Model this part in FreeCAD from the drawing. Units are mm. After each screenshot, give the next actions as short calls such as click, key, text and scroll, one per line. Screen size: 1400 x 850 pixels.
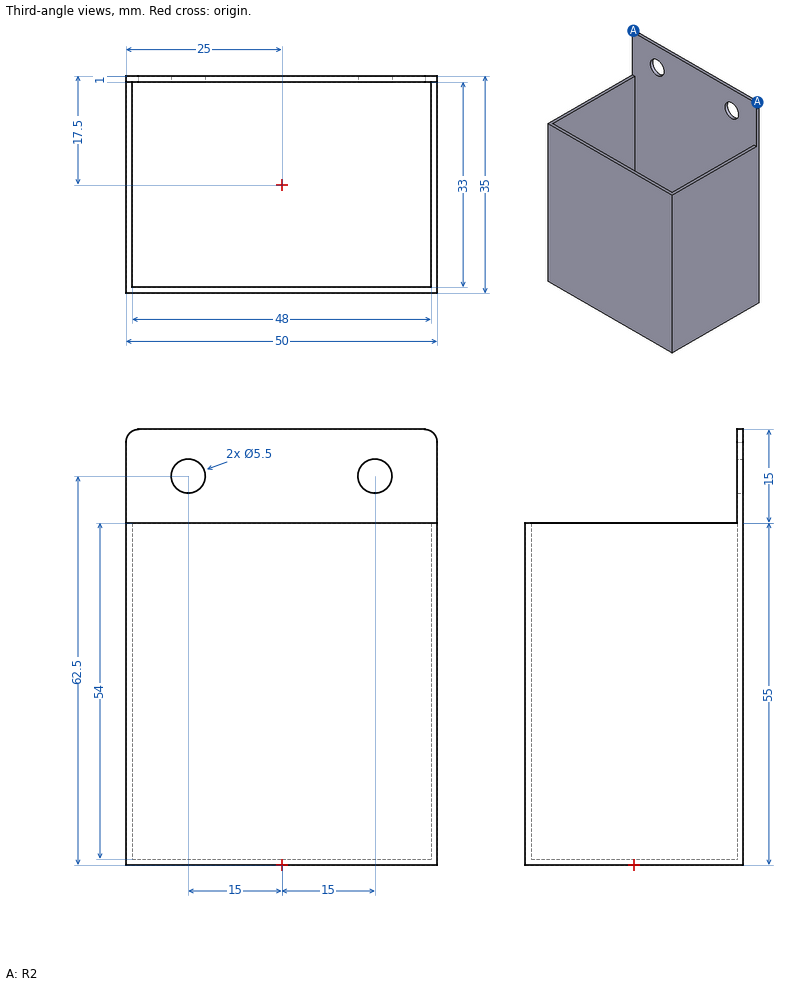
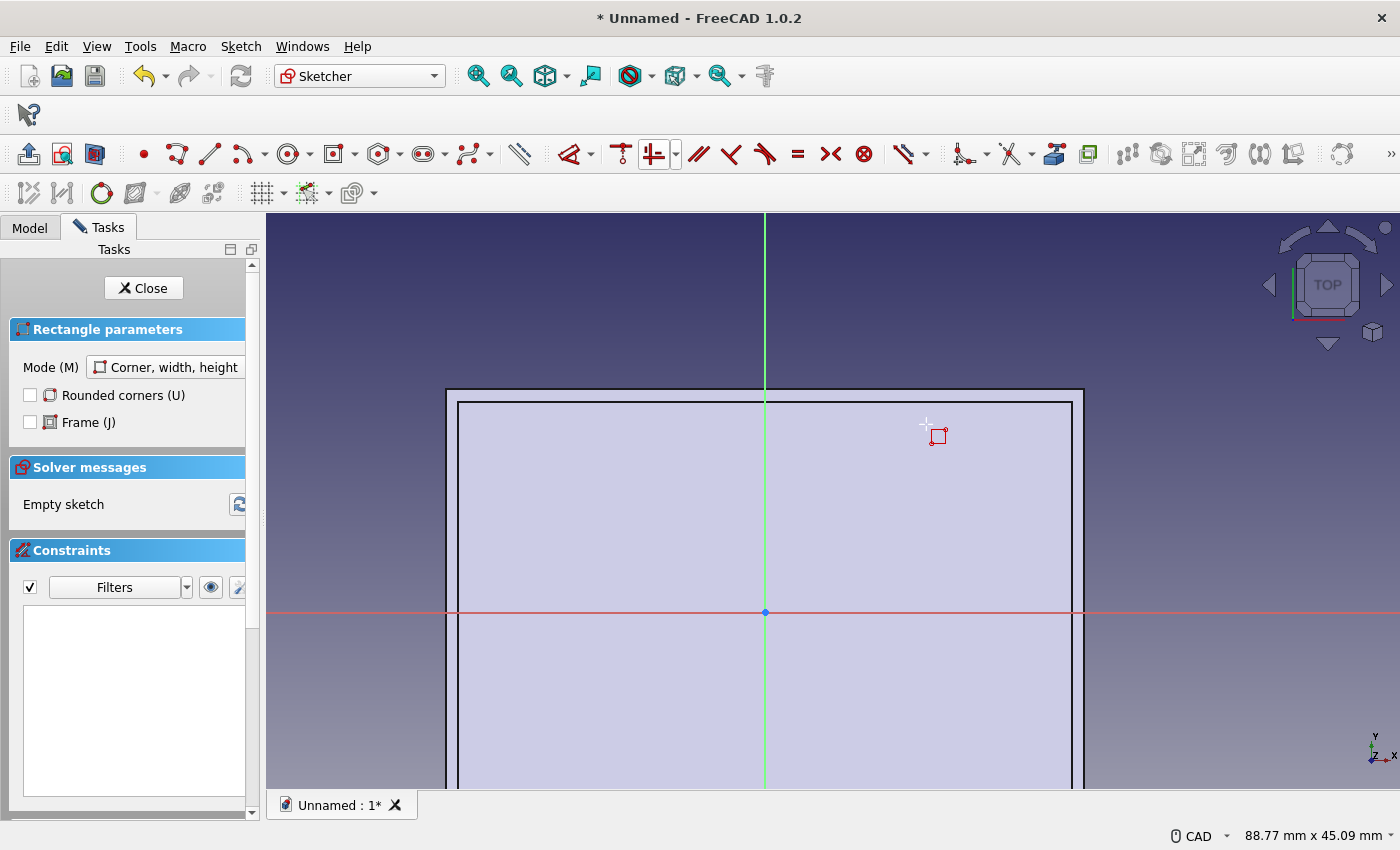
scroll(446, 389, up, 2)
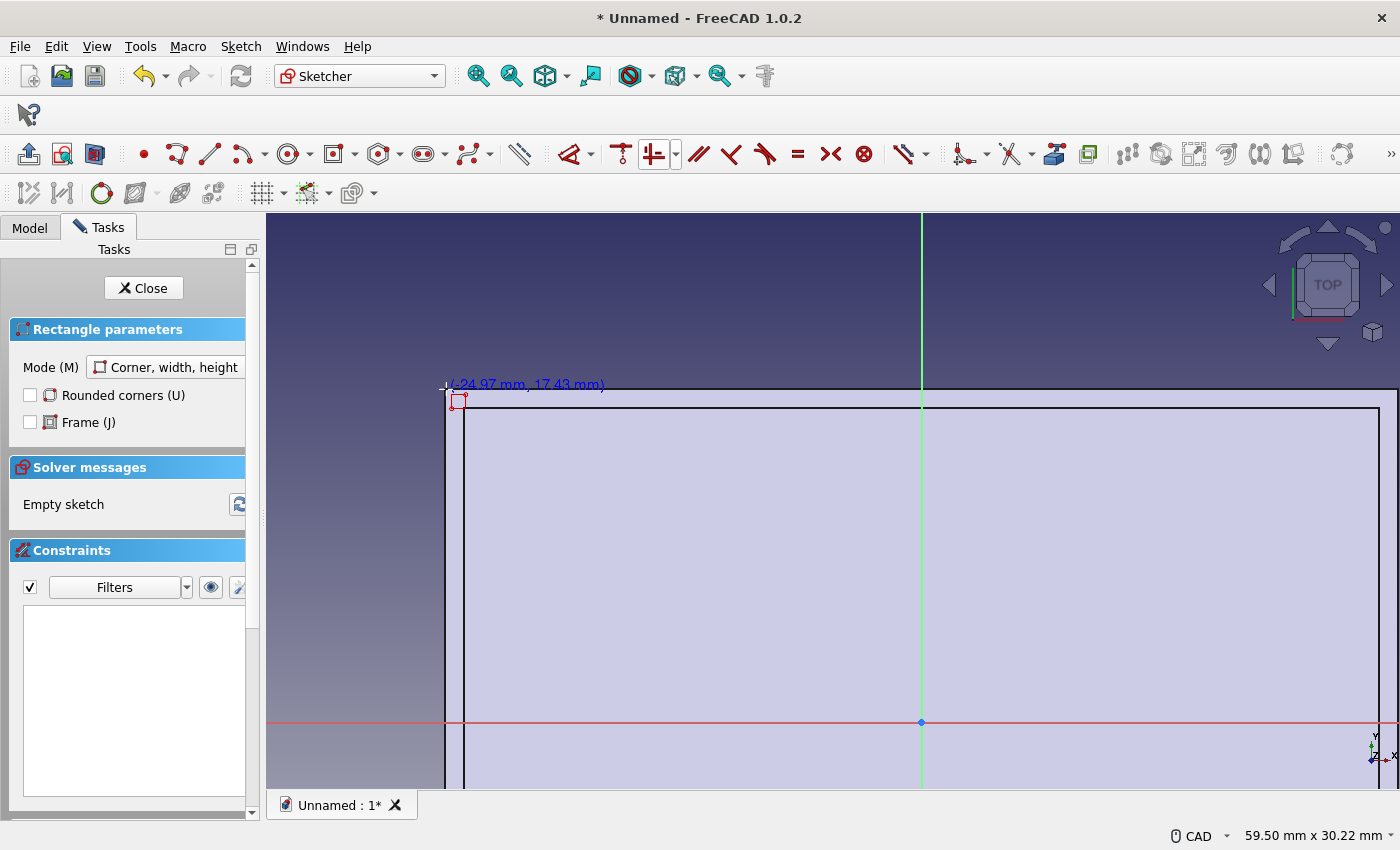
click(445, 389)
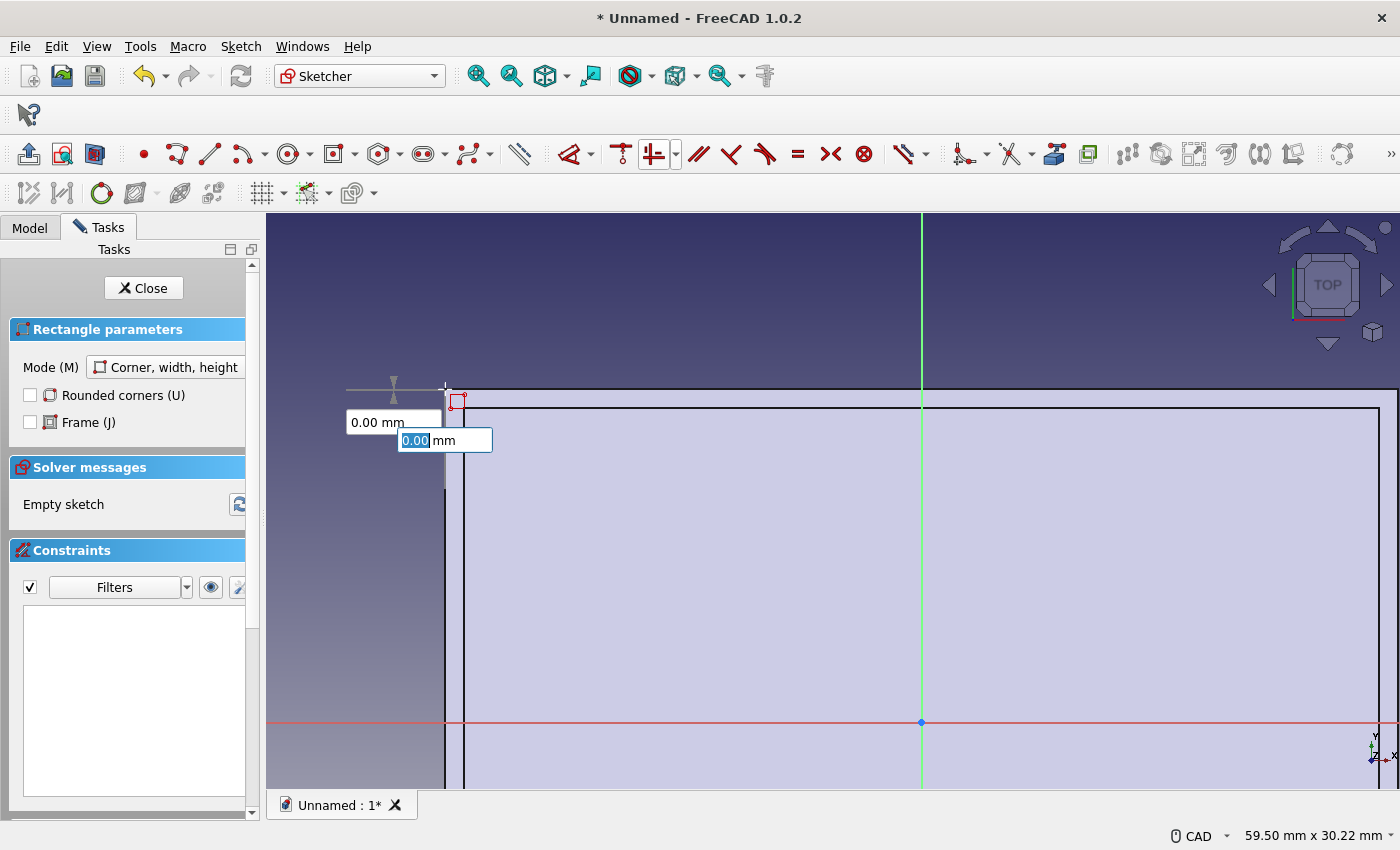
scroll(445, 390, down, 2)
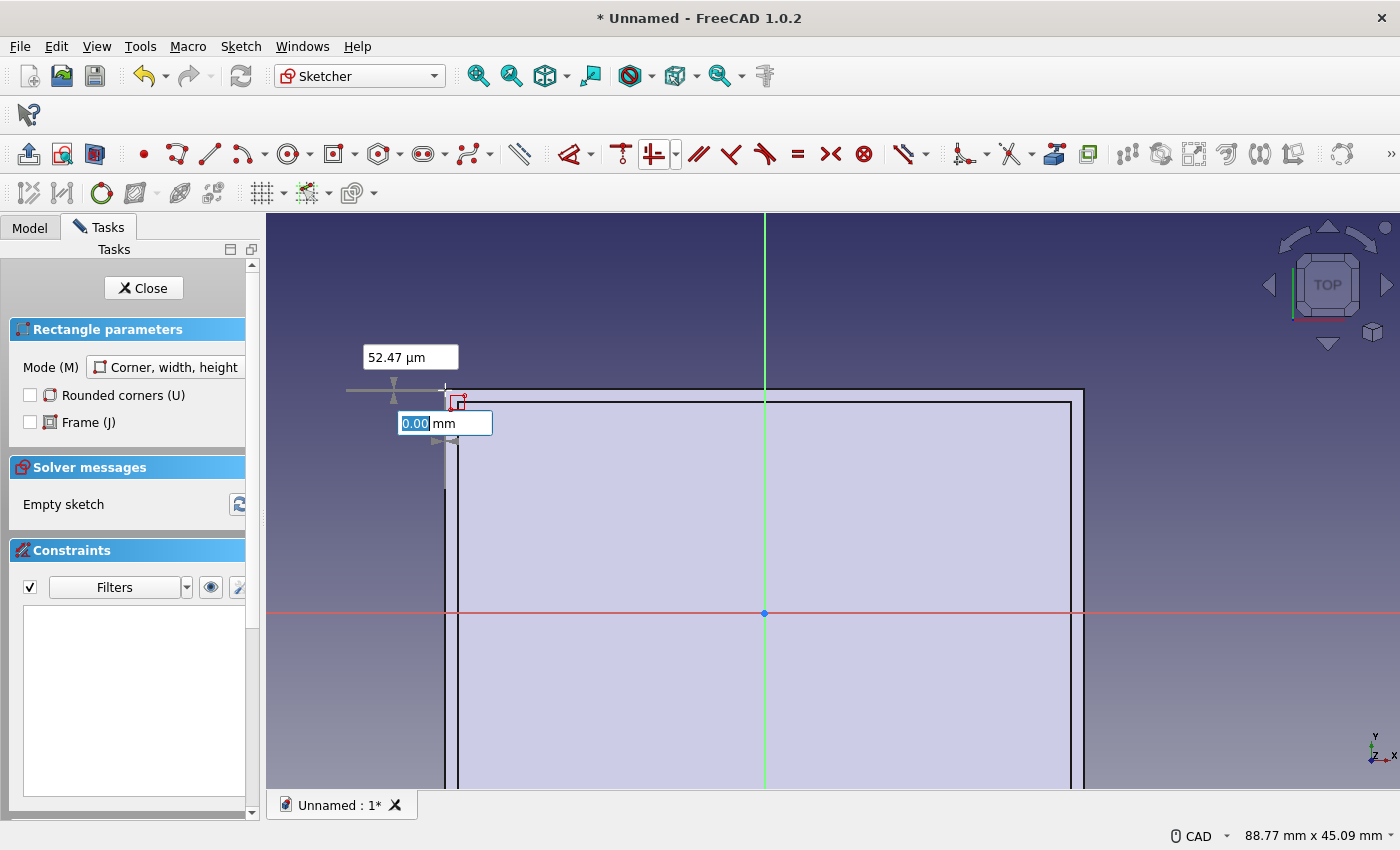
click(1084, 402)
key(Escape)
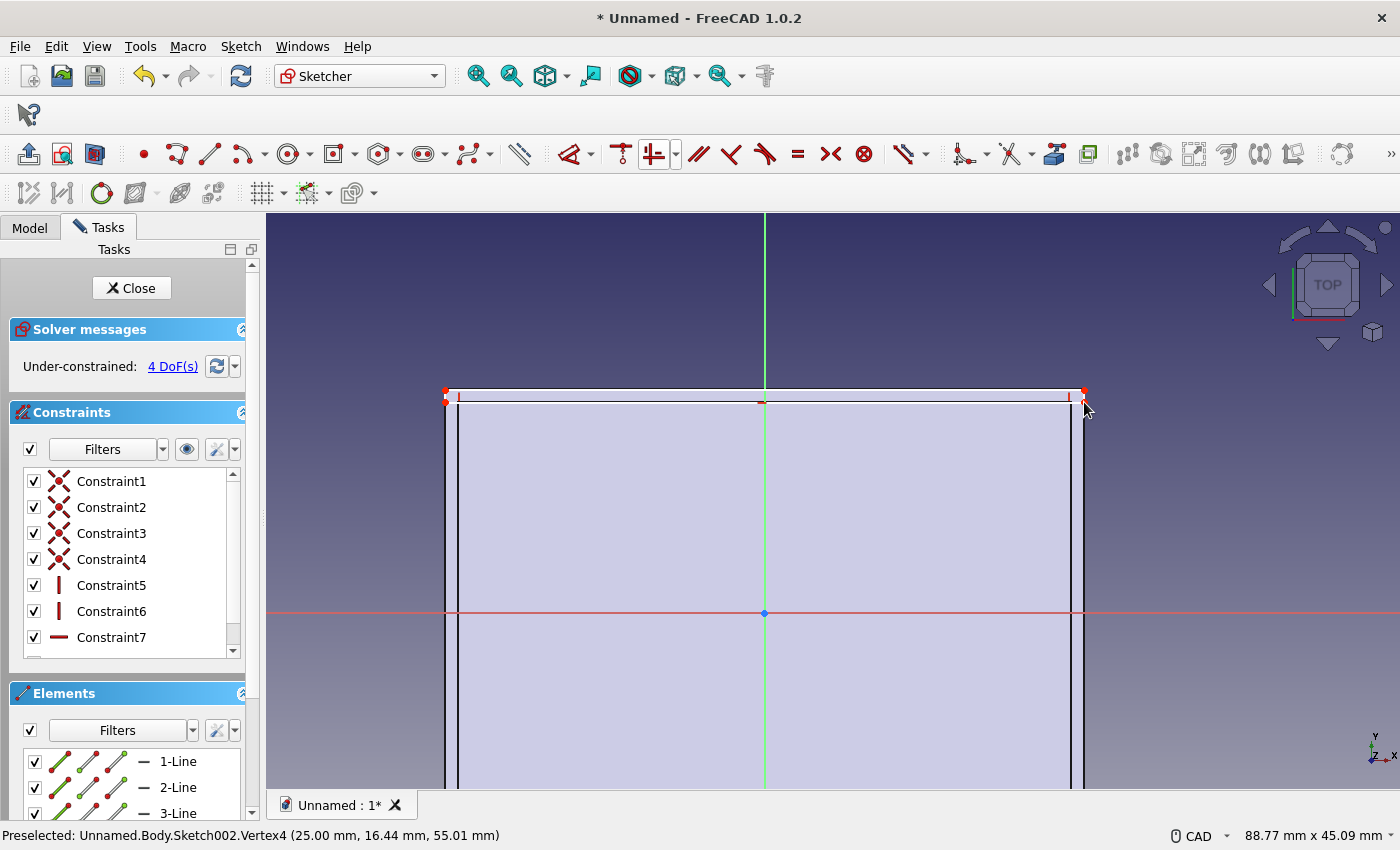
key(d)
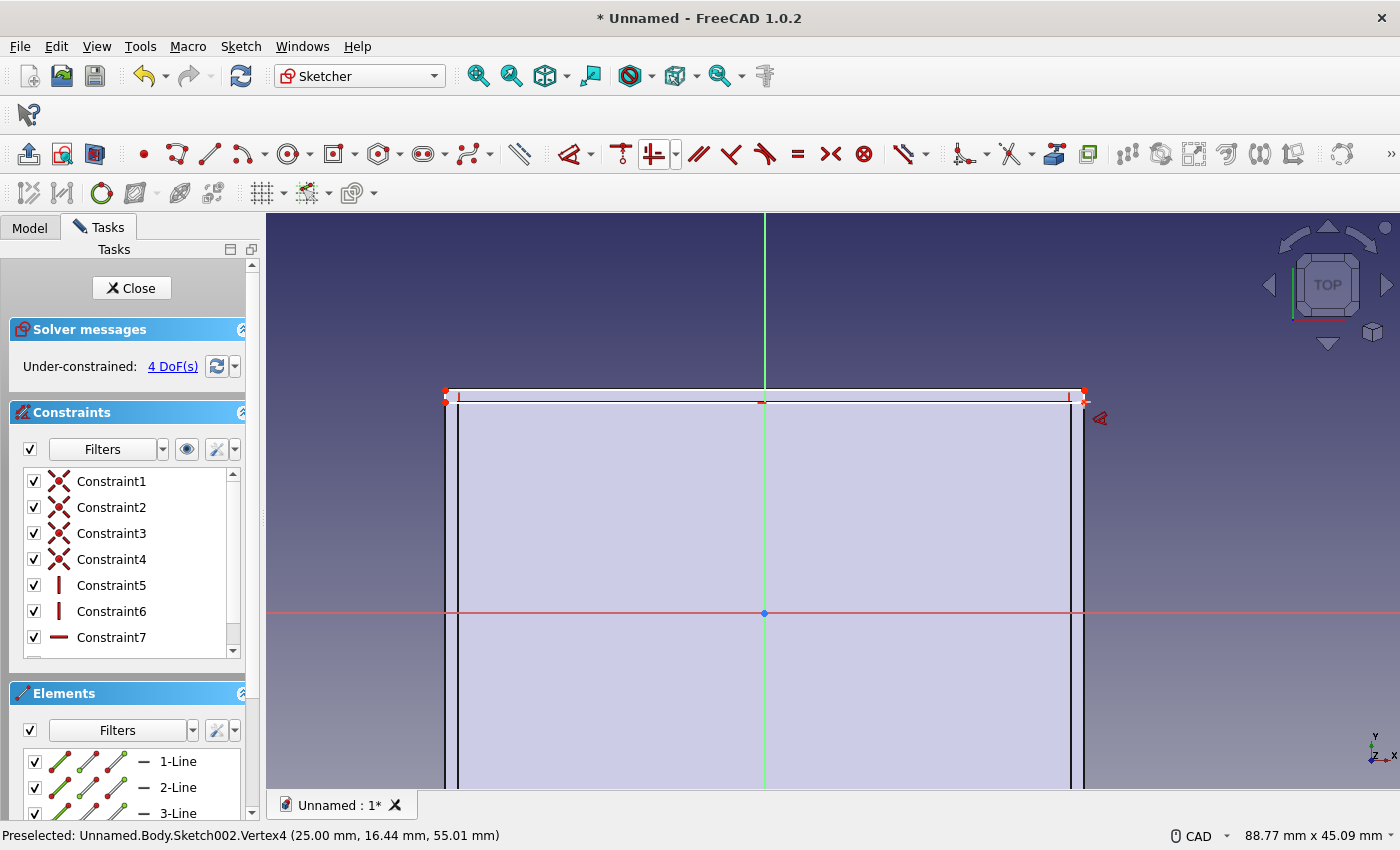
scroll(445, 397, up, 6)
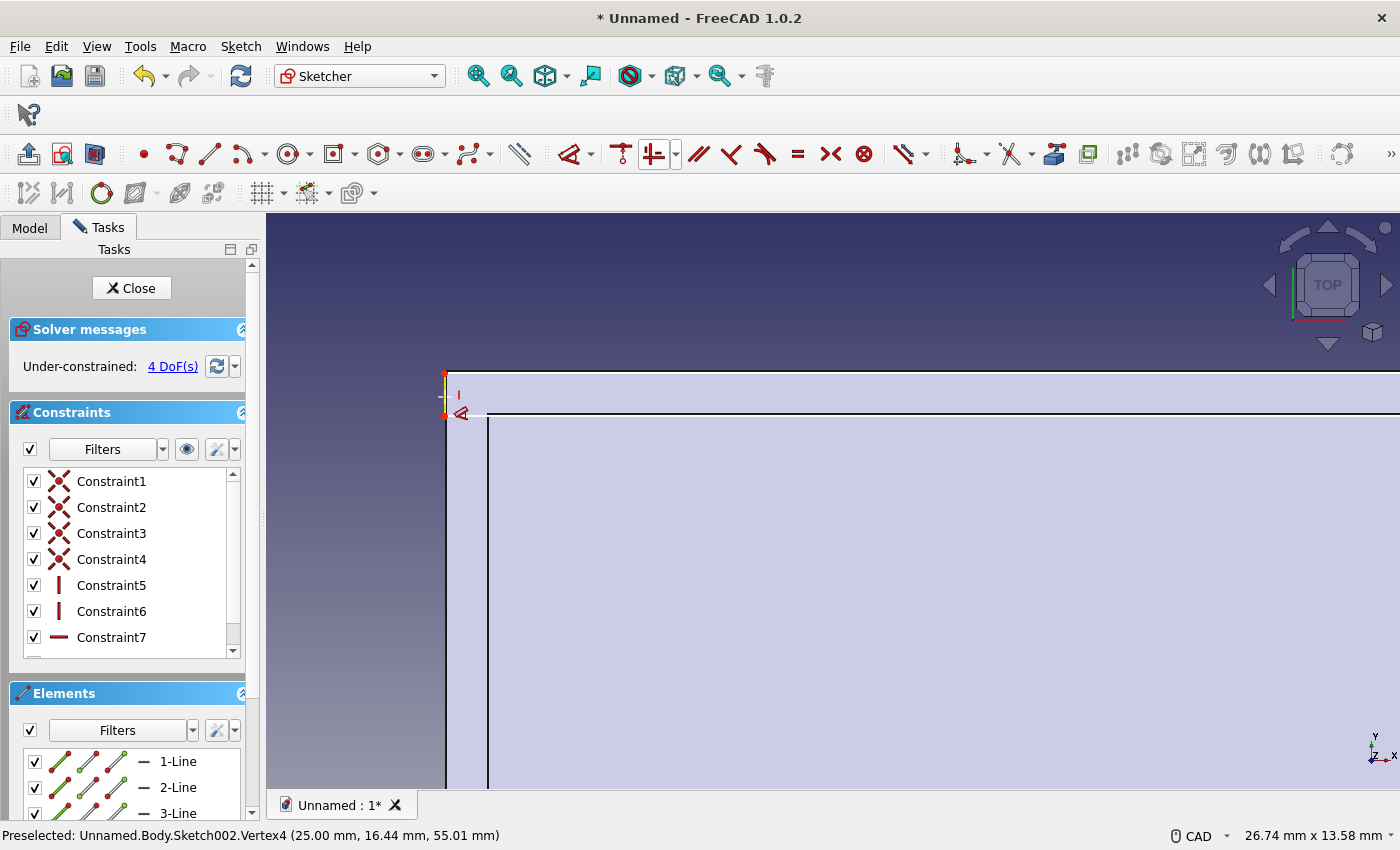
click(445, 395)
click(411, 395)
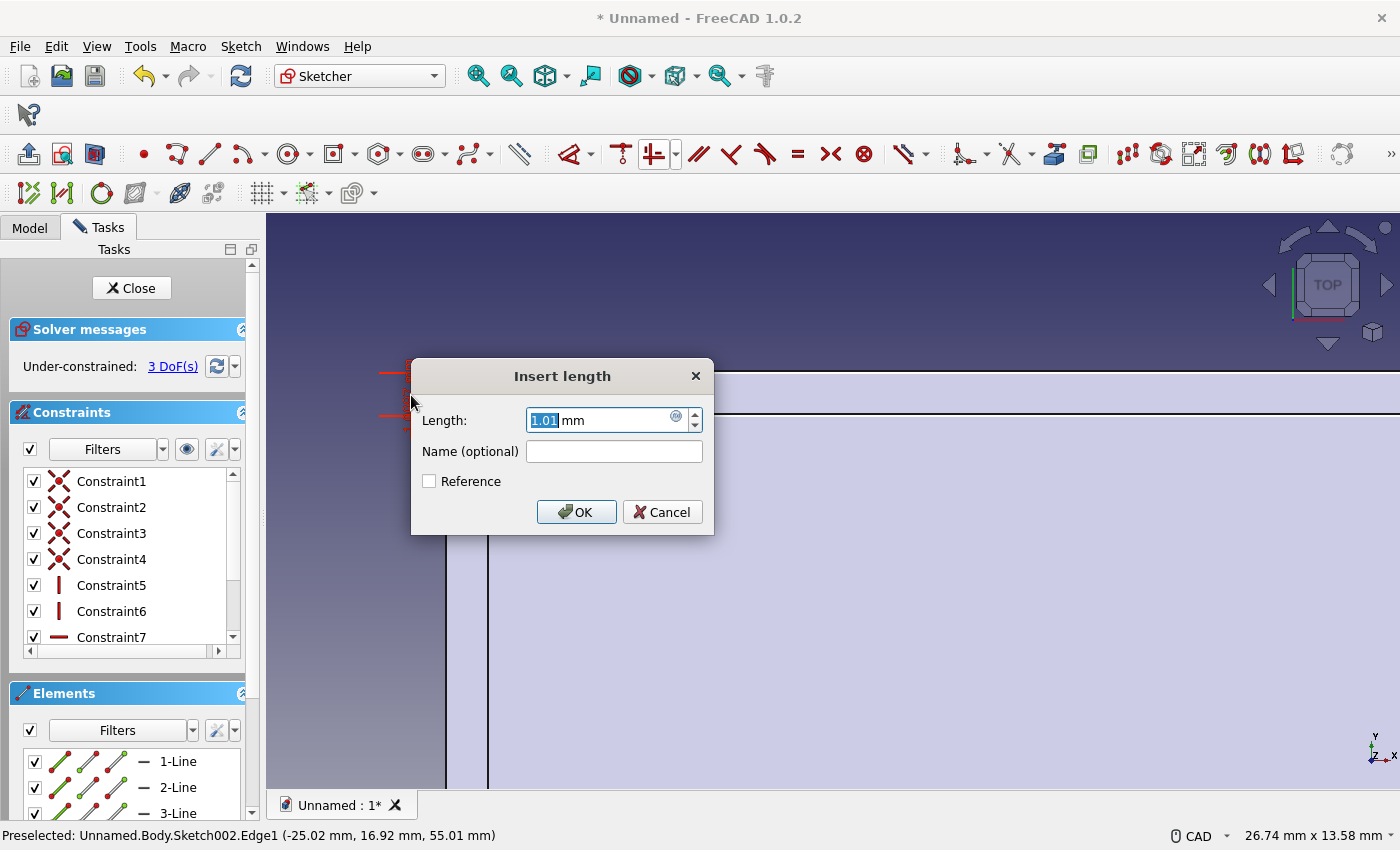
text(1)
key(Return)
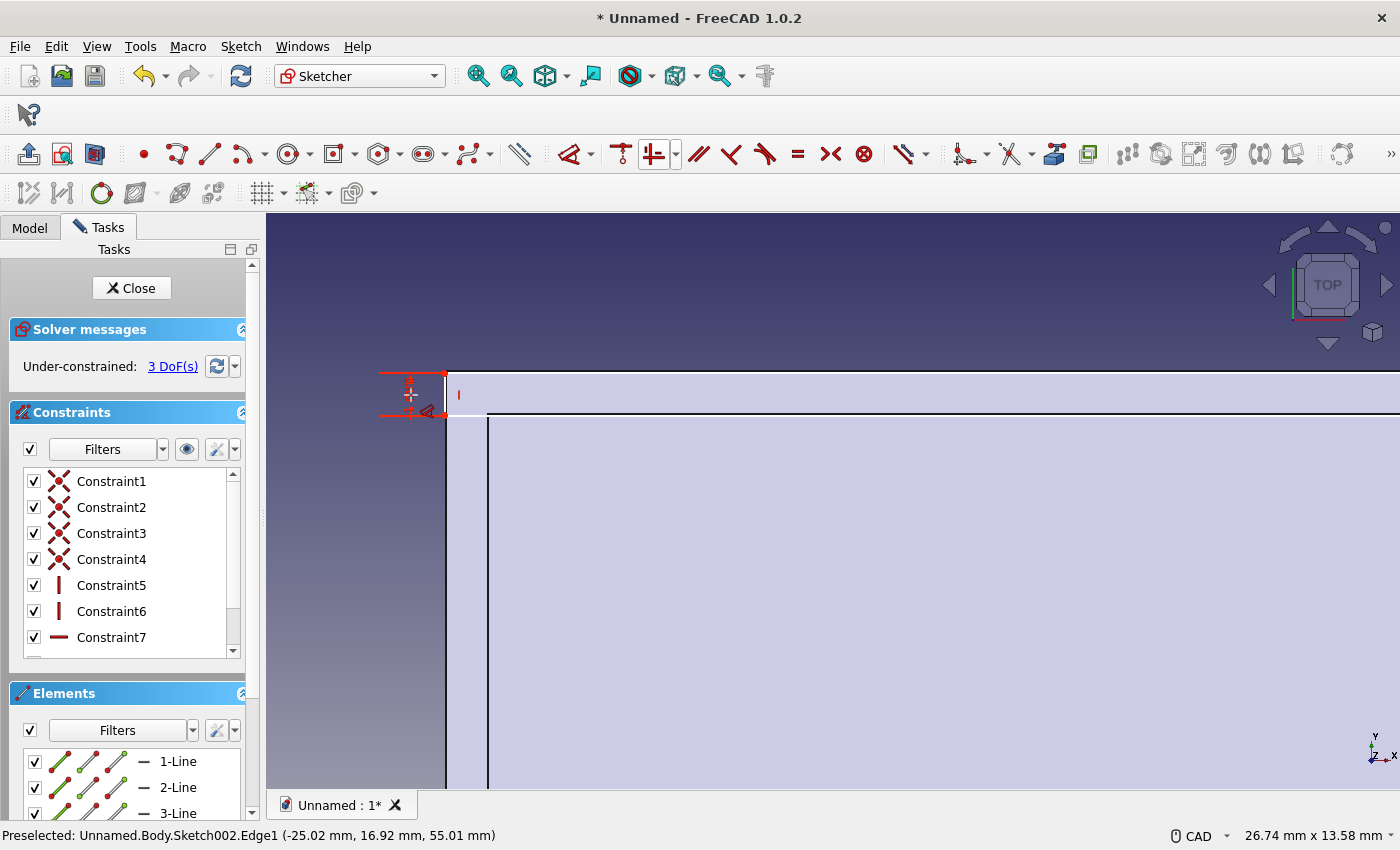
click(1081, 416)
click(840, 450)